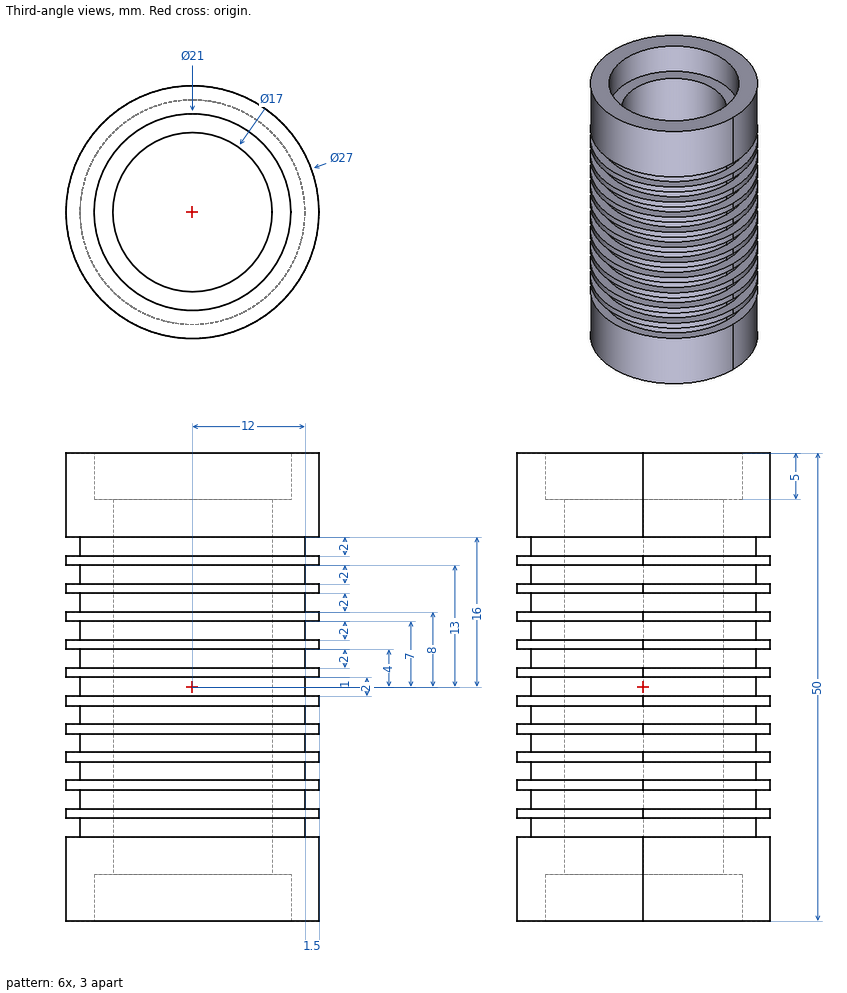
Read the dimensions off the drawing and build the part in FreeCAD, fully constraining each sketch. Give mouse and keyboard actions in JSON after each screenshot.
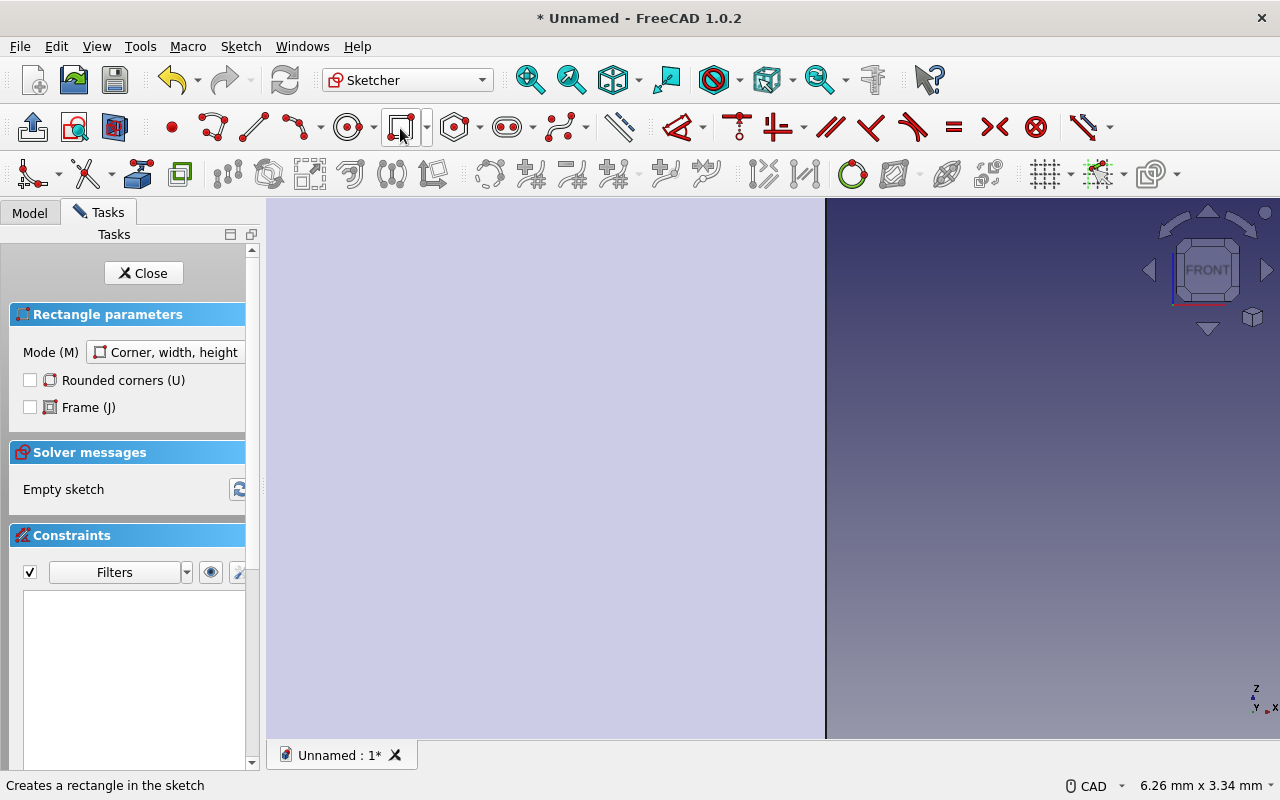
{"action": "left_click", "coordinate": [583, 306]}
{"action": "mouse_move", "coordinate": [826, 630]}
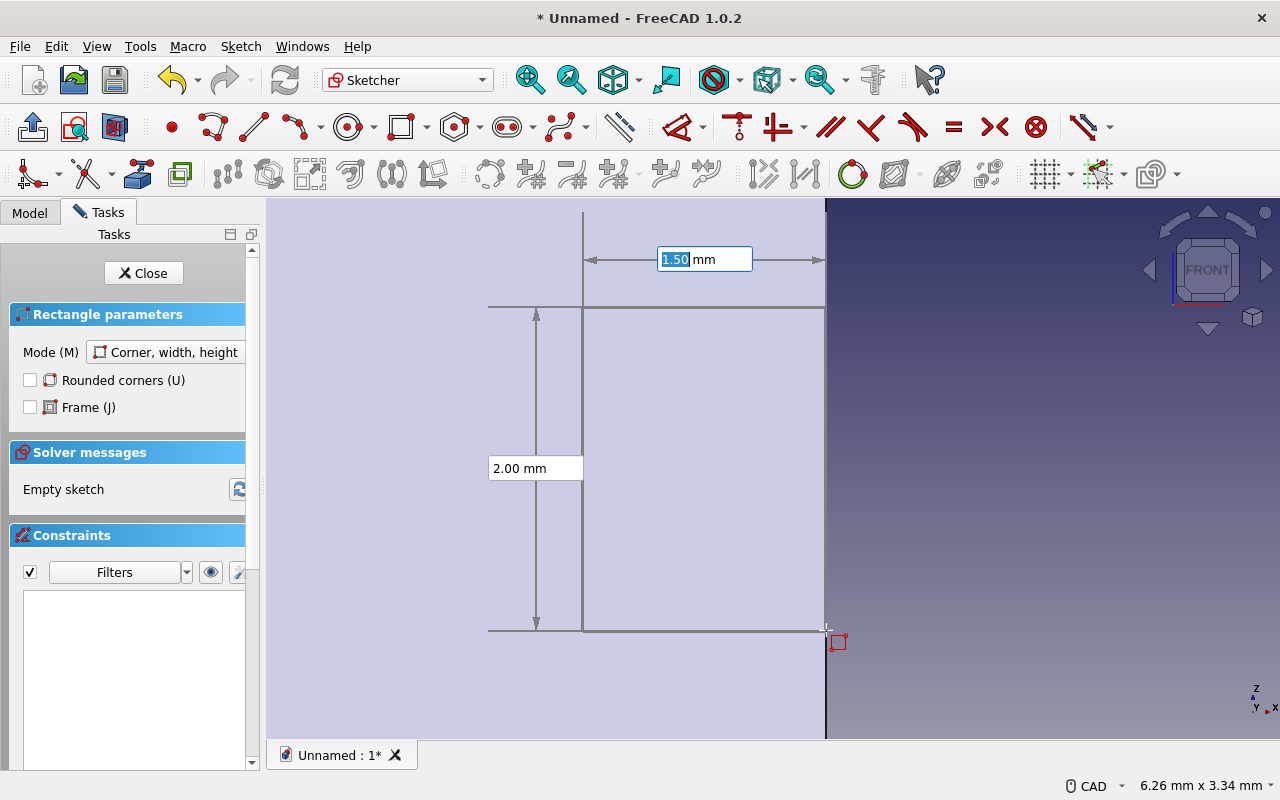
{"action": "type", "text": "1.5"}
{"action": "key", "text": "Tab"}
{"action": "type", "text": "2"}
{"action": "key", "text": "Return"}
{"action": "key", "text": "Escape"}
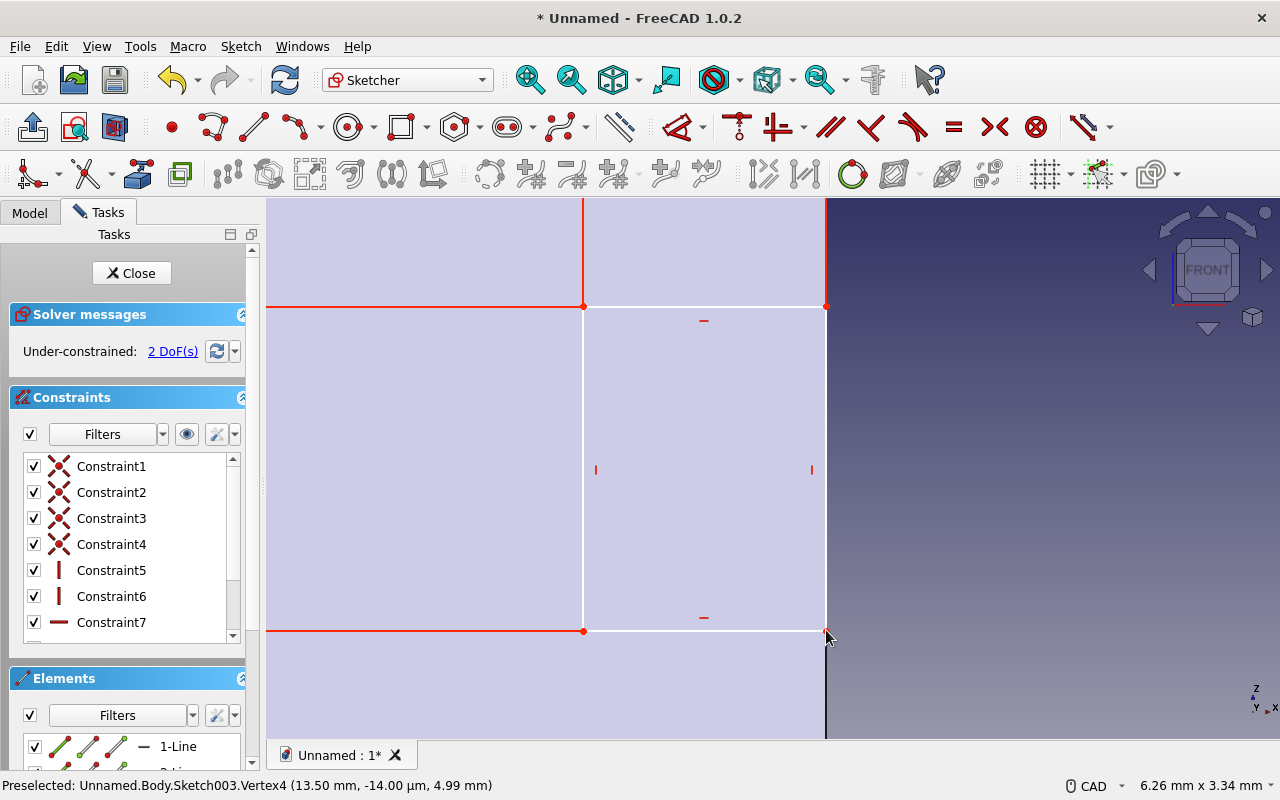
{"action": "left_click", "coordinate": [676, 128]}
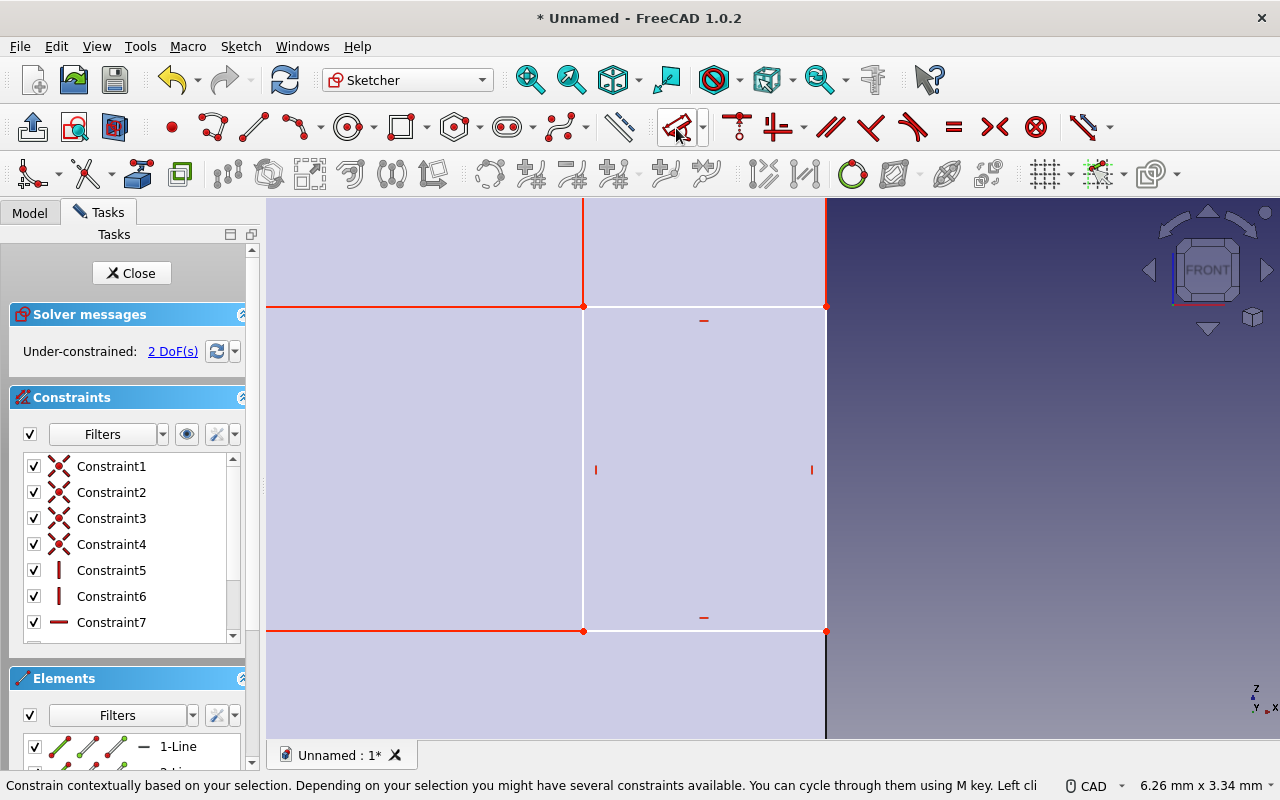
{"action": "left_click", "coordinate": [583, 307]}
{"action": "left_click", "coordinate": [617, 509]}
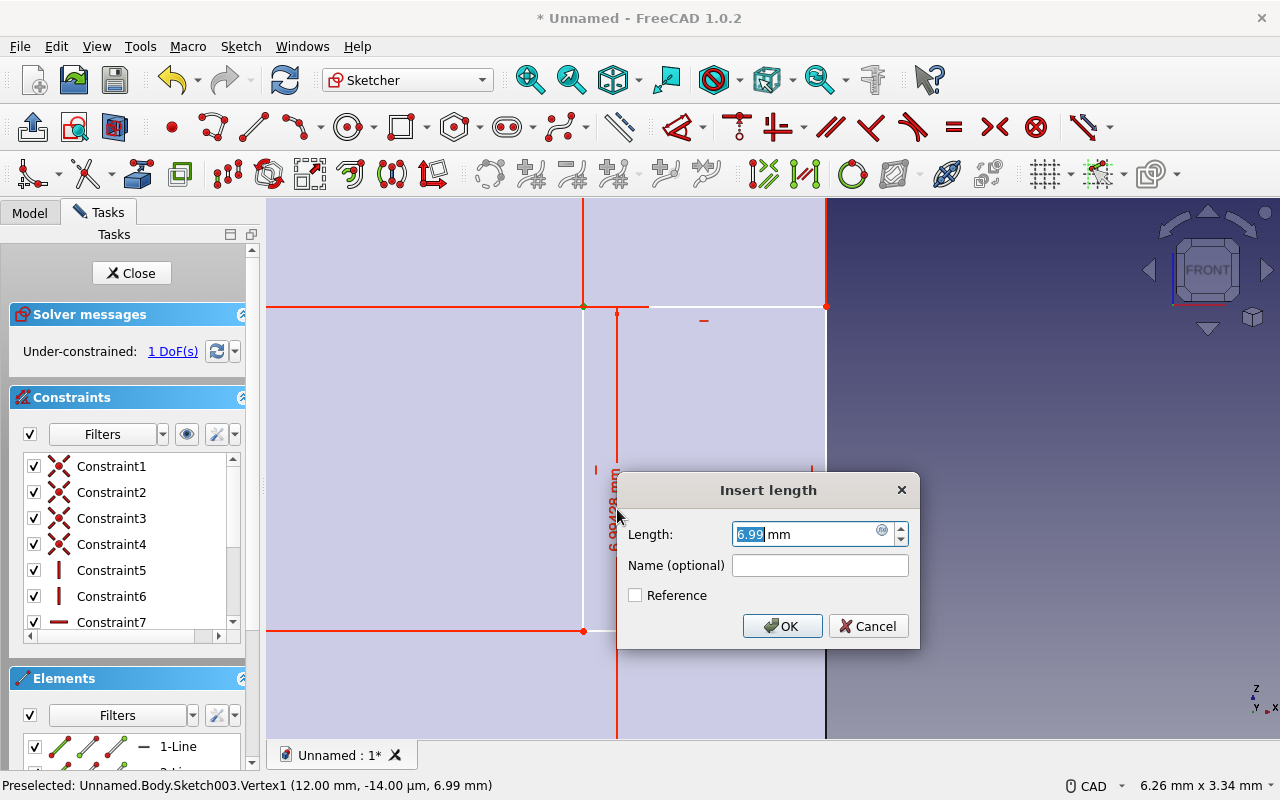
{"action": "type", "text": "7"}
{"action": "key", "text": "Return"}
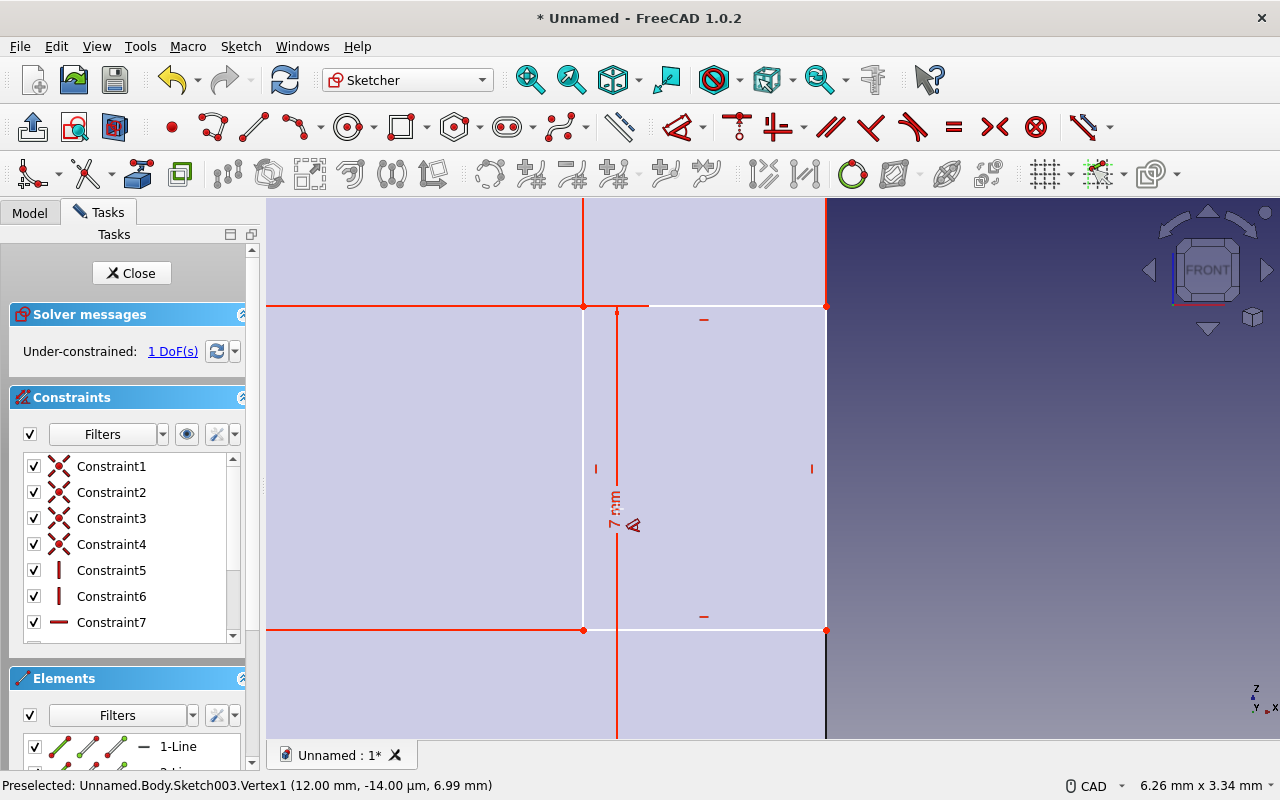
{"action": "left_click", "coordinate": [583, 306]}
{"action": "left_click", "coordinate": [438, 272]}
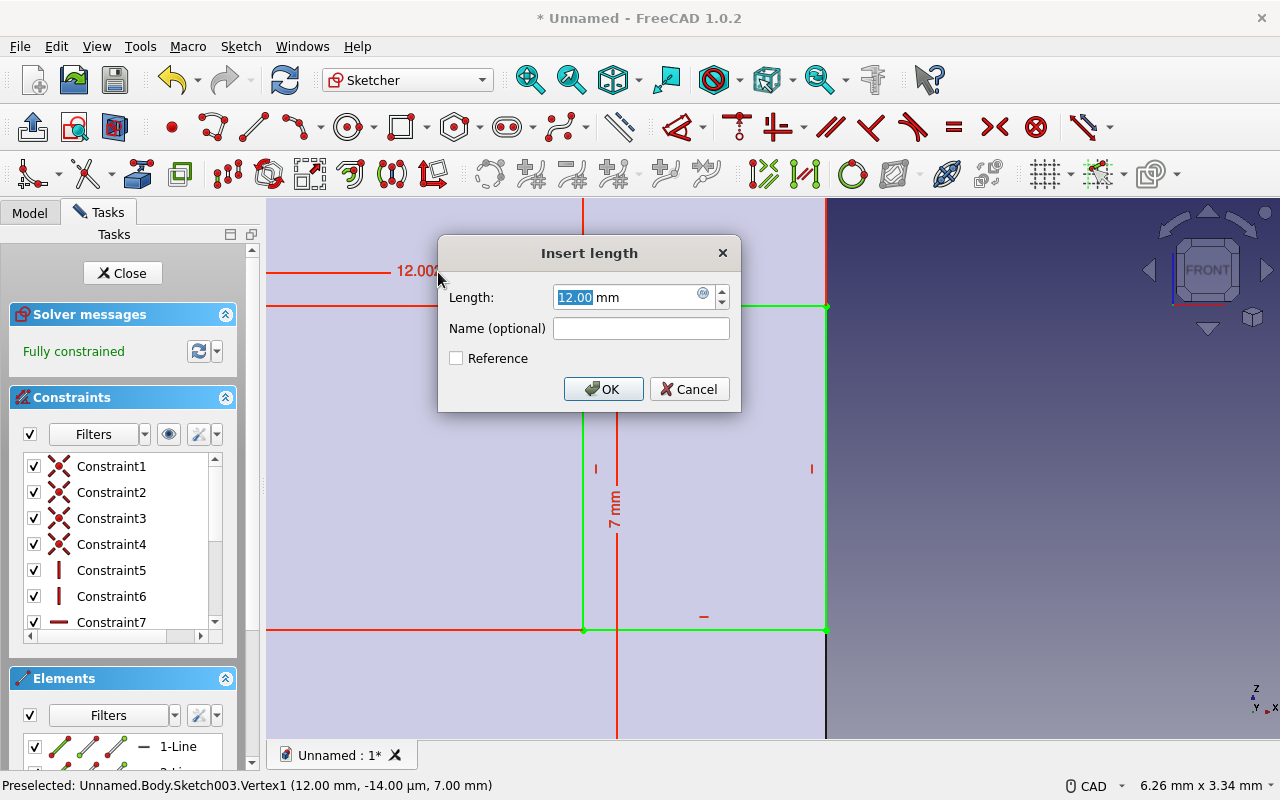
{"action": "type", "text": "12"}
{"action": "key", "text": "Return"}
{"action": "key", "text": "Escape"}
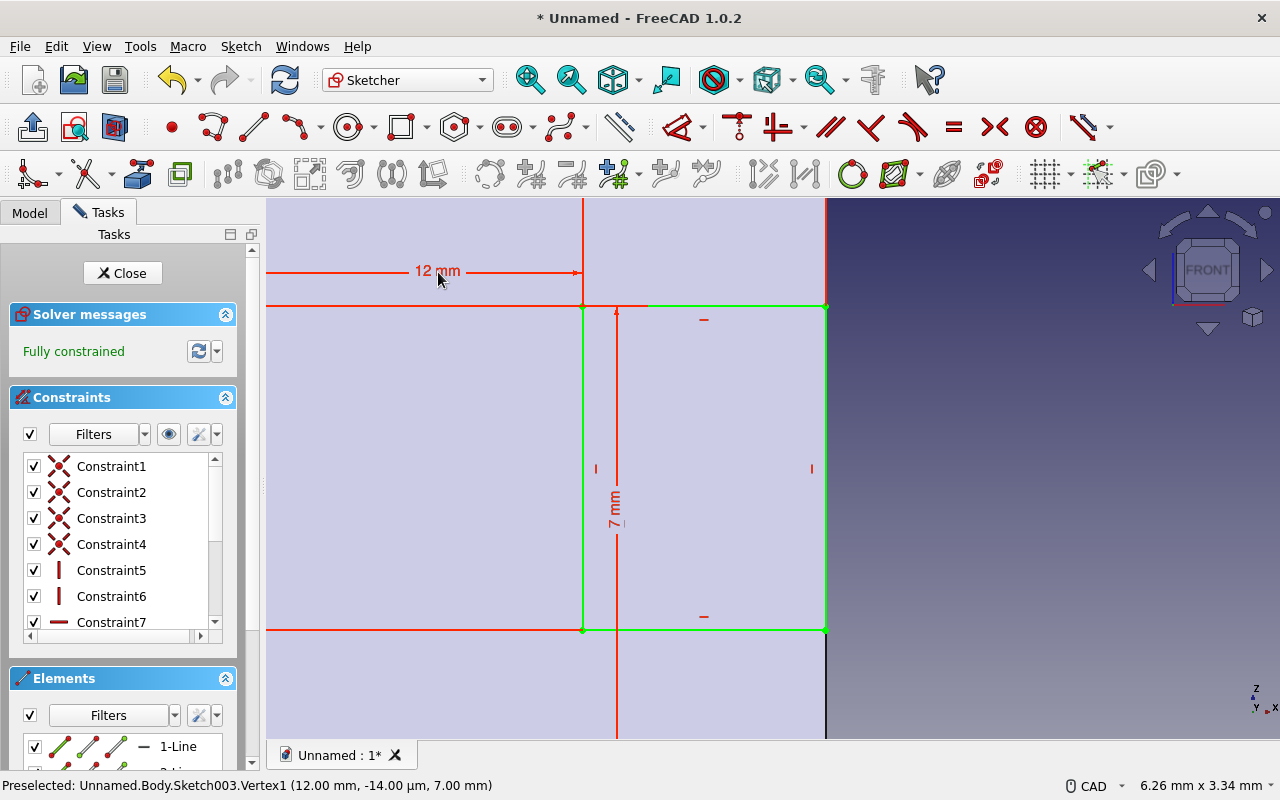
{"action": "left_click", "coordinate": [123, 273]}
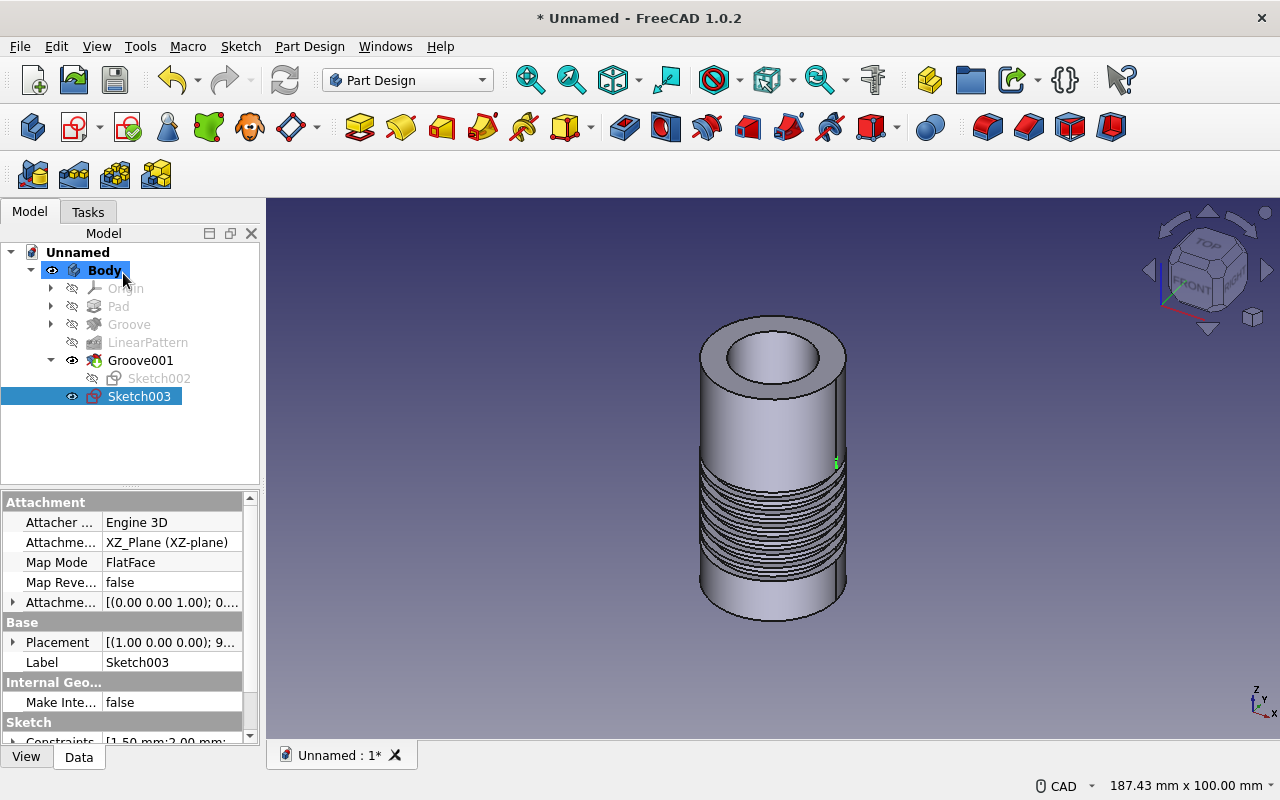
{"action": "left_click", "coordinate": [707, 128]}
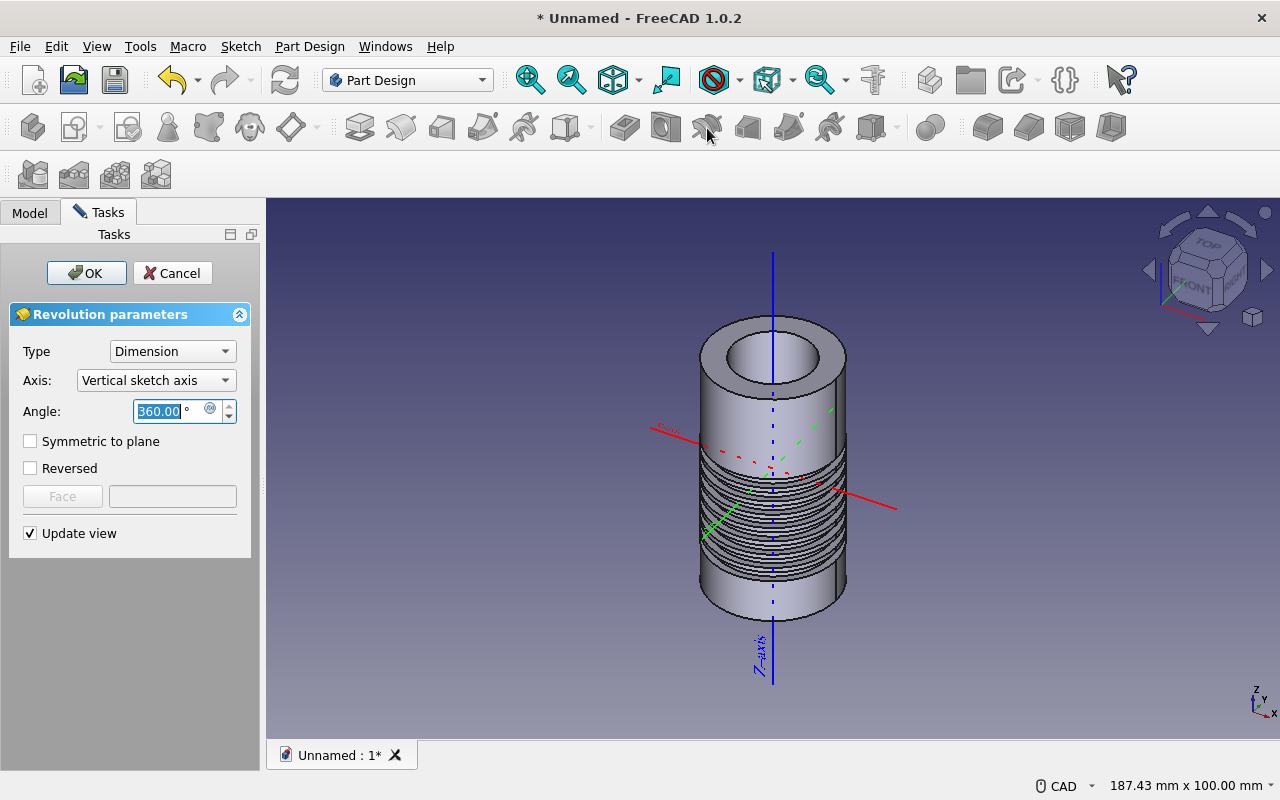
{"action": "left_click", "coordinate": [87, 273]}